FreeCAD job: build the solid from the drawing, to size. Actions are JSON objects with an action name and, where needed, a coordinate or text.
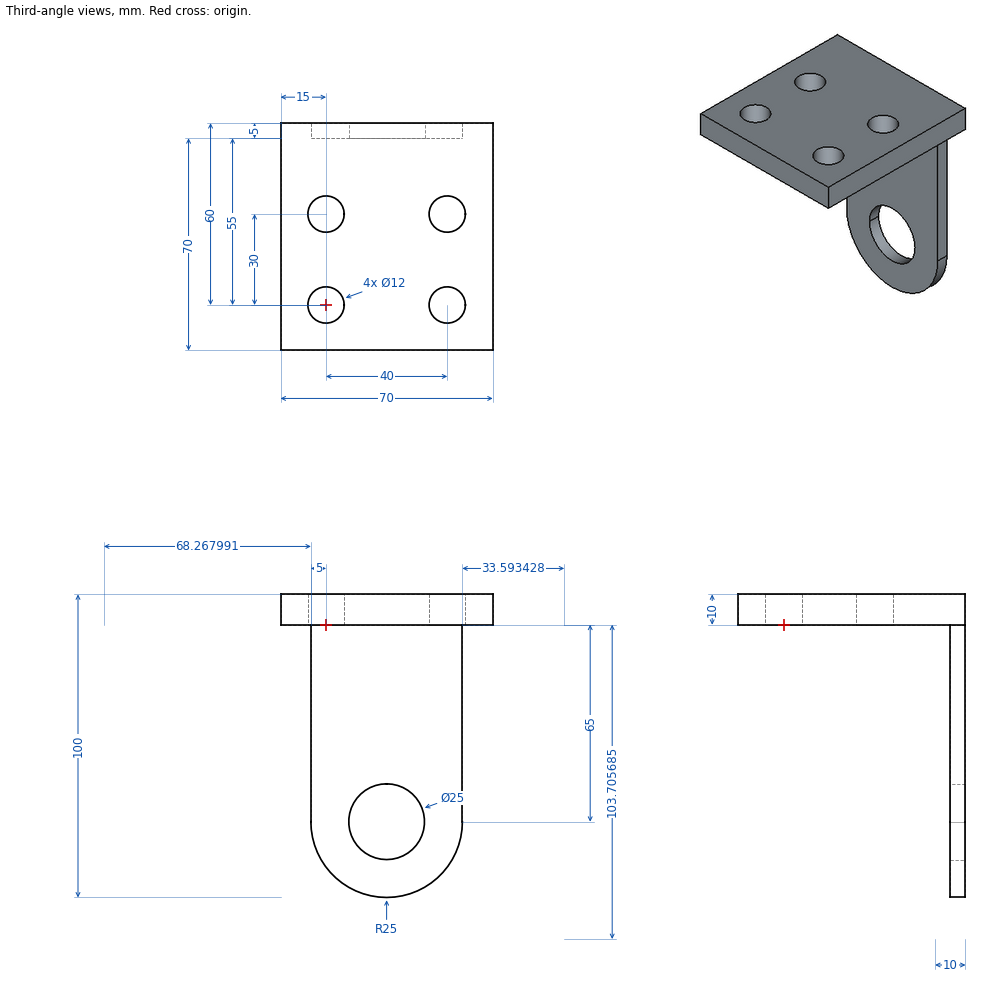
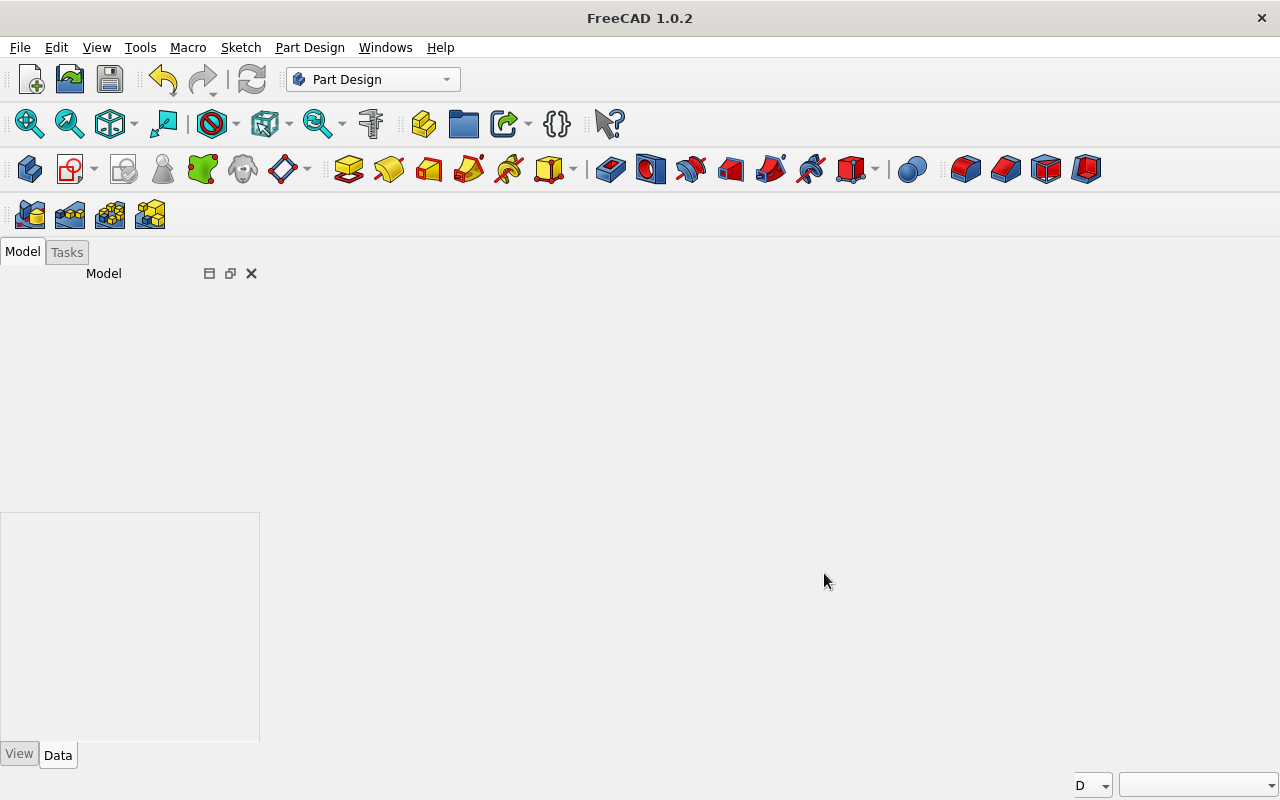
{"action": "left_click", "coordinate": [30, 80]}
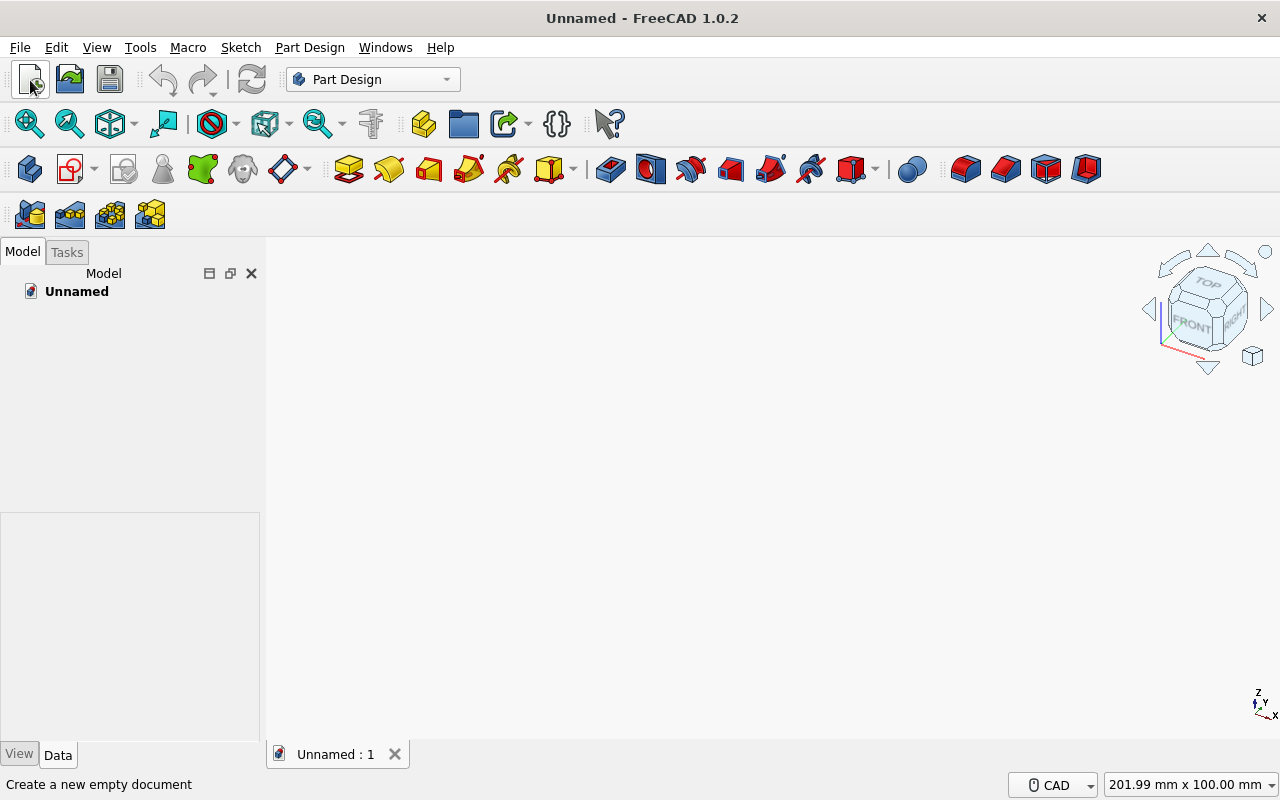
{"action": "left_click", "coordinate": [70, 170]}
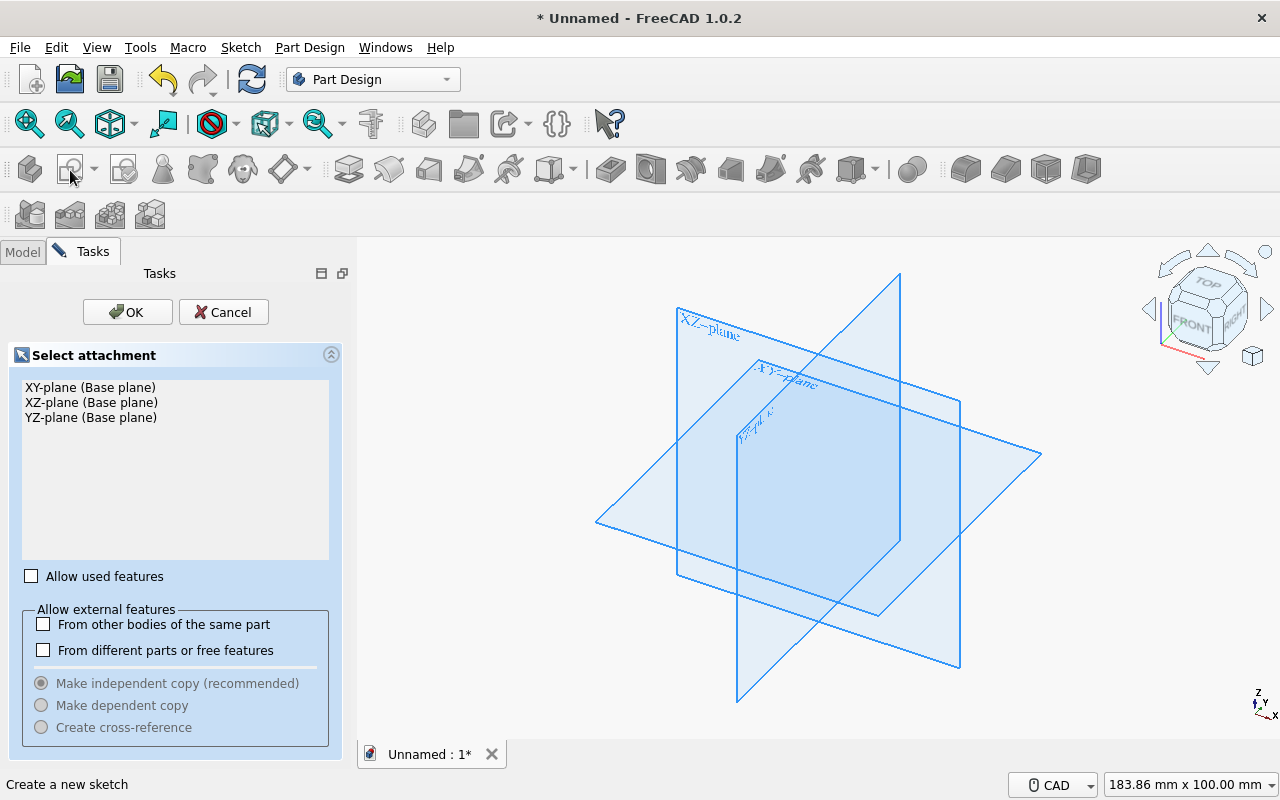
{"action": "left_click", "coordinate": [82, 388]}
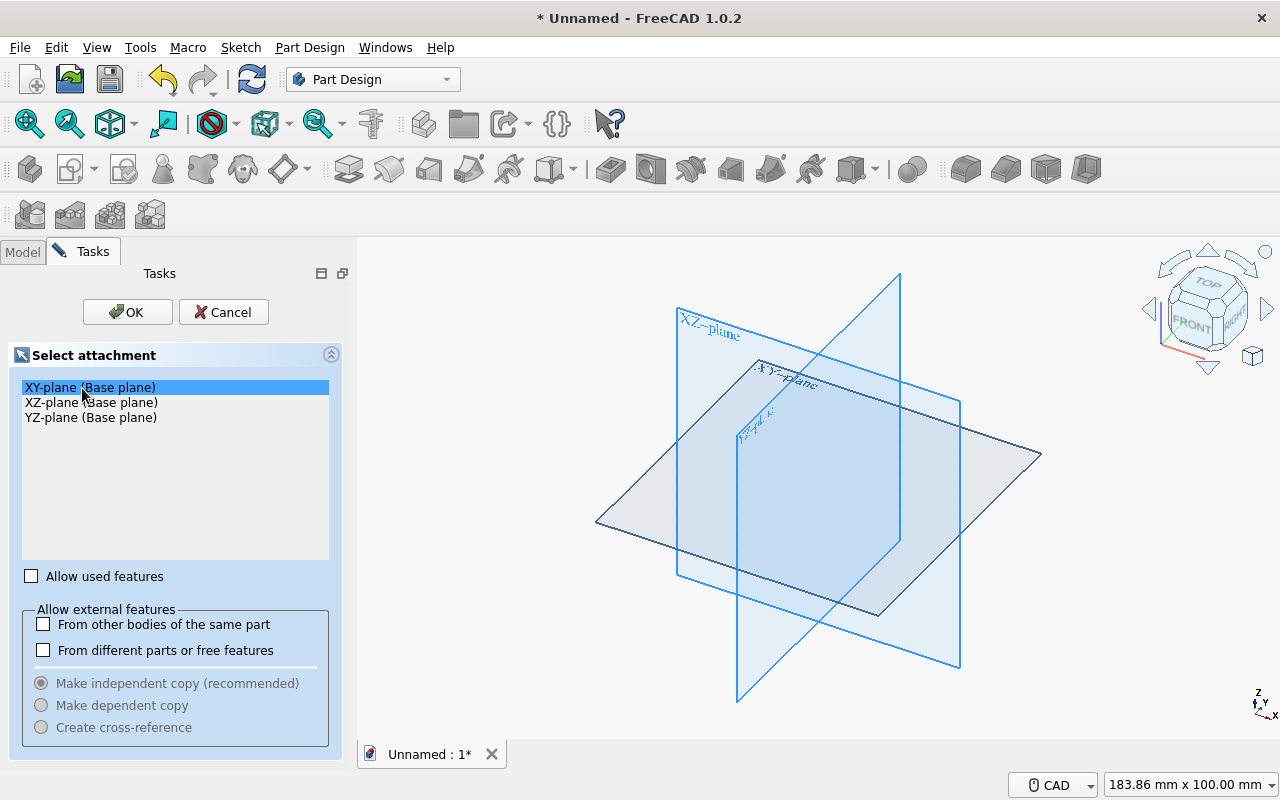
{"action": "left_click", "coordinate": [128, 312]}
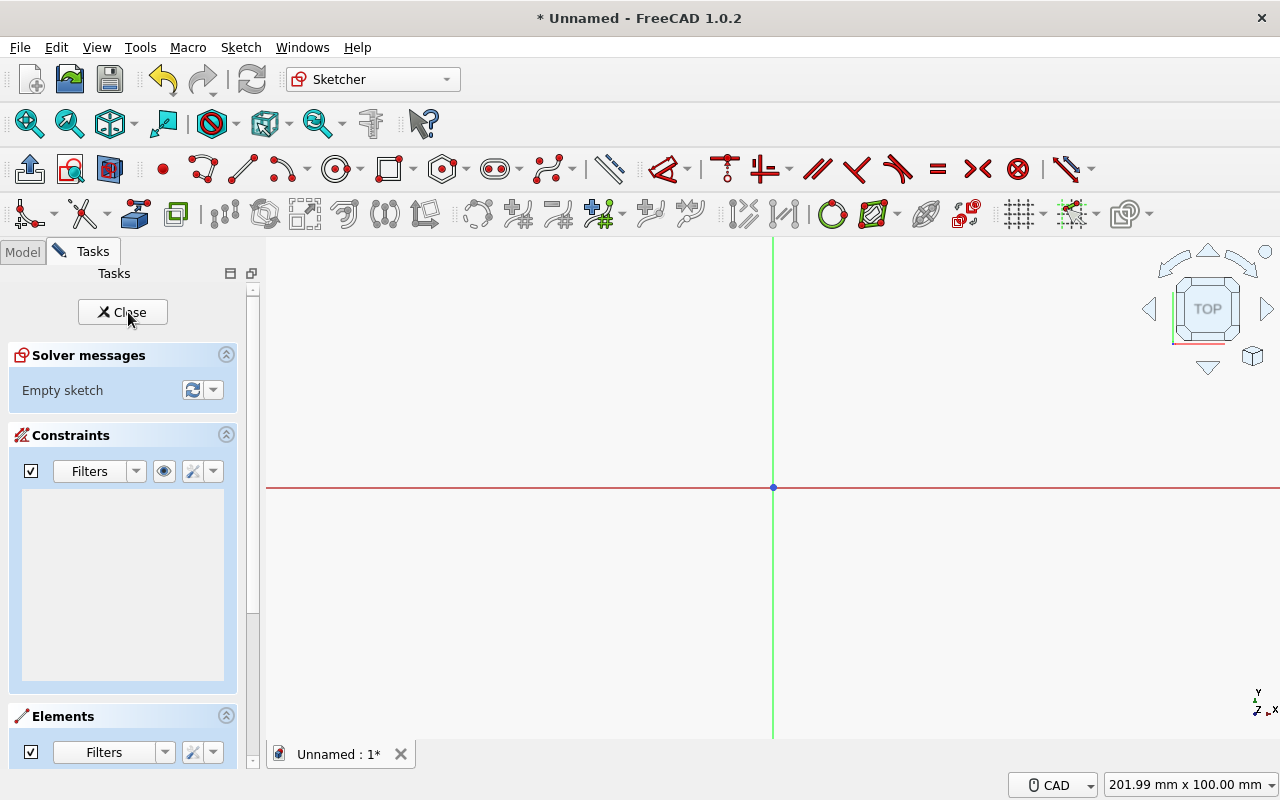
{"action": "scroll", "coordinate": [294, 711], "scroll_direction": "down", "scroll_amount": 1}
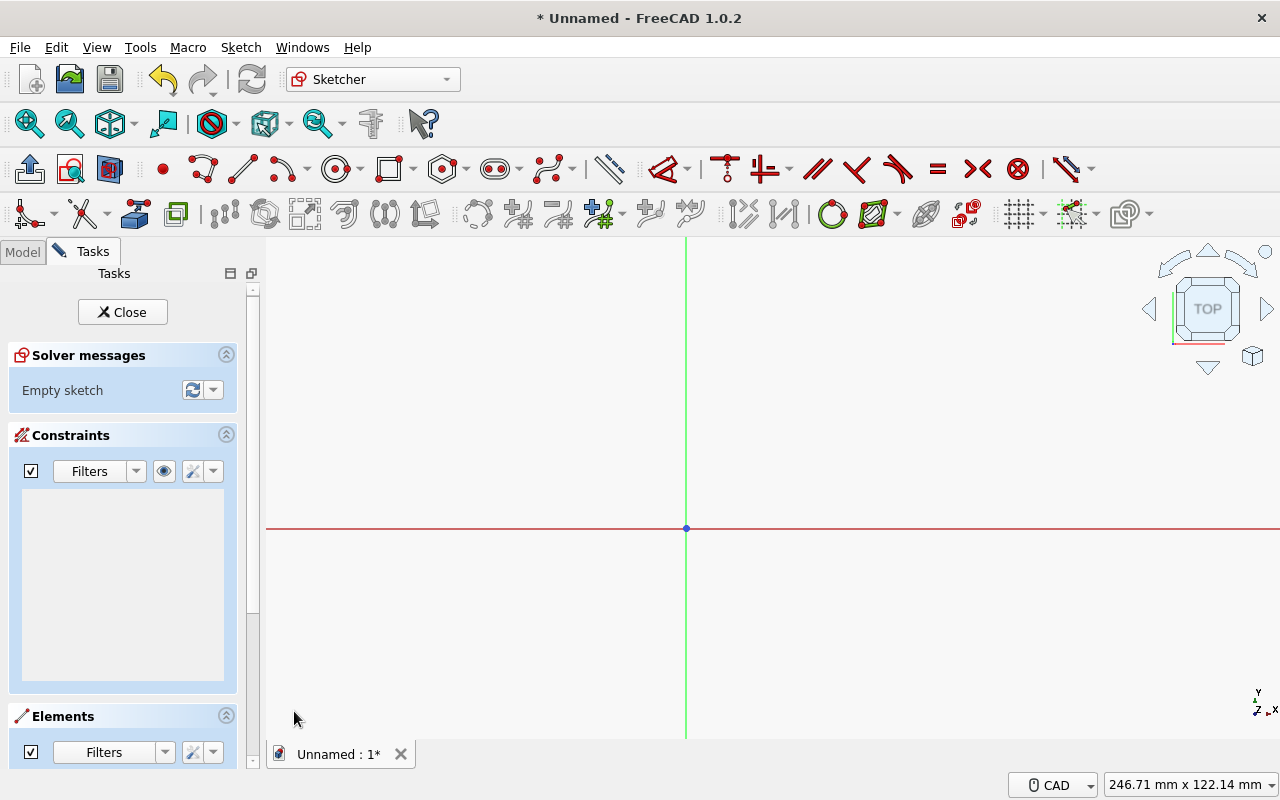
{"action": "left_click", "coordinate": [390, 170]}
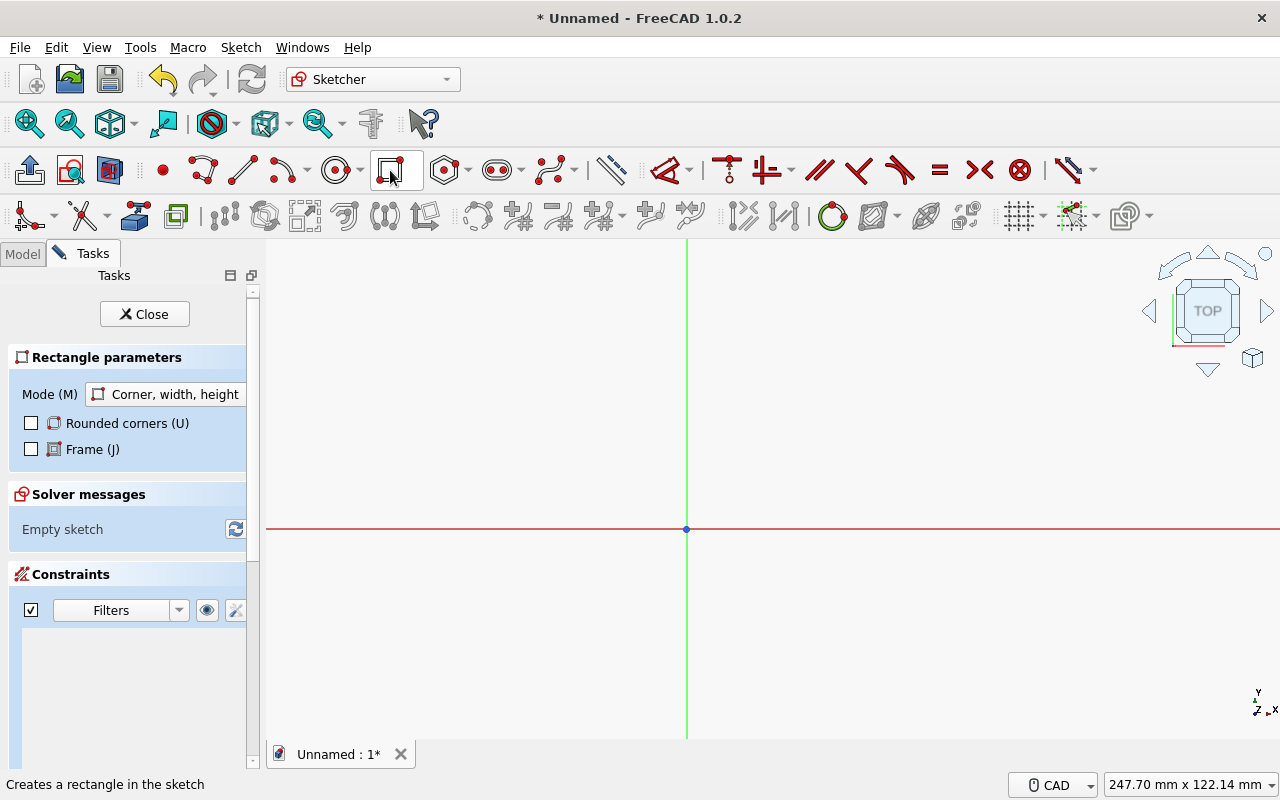
{"action": "left_click", "coordinate": [625, 304]}
{"action": "left_click", "coordinate": [912, 591]}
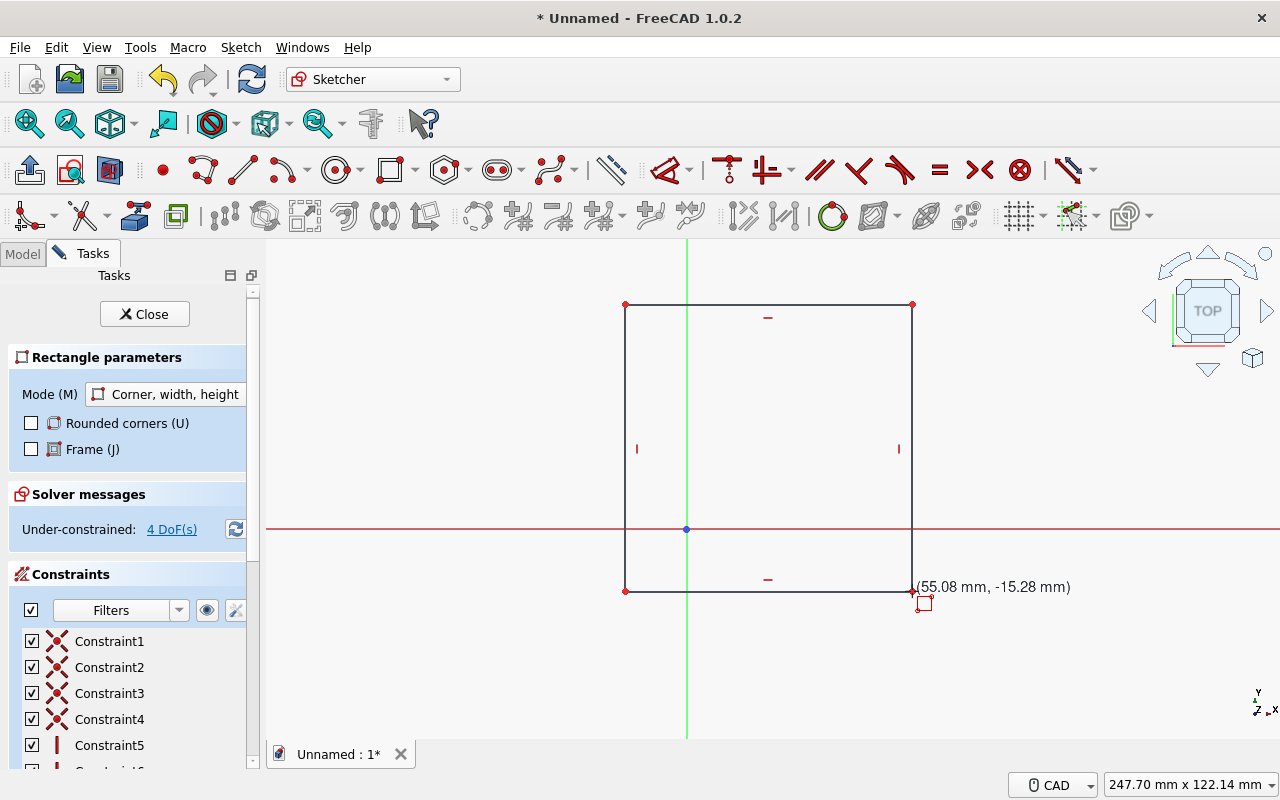
{"action": "left_click", "coordinate": [336, 170]}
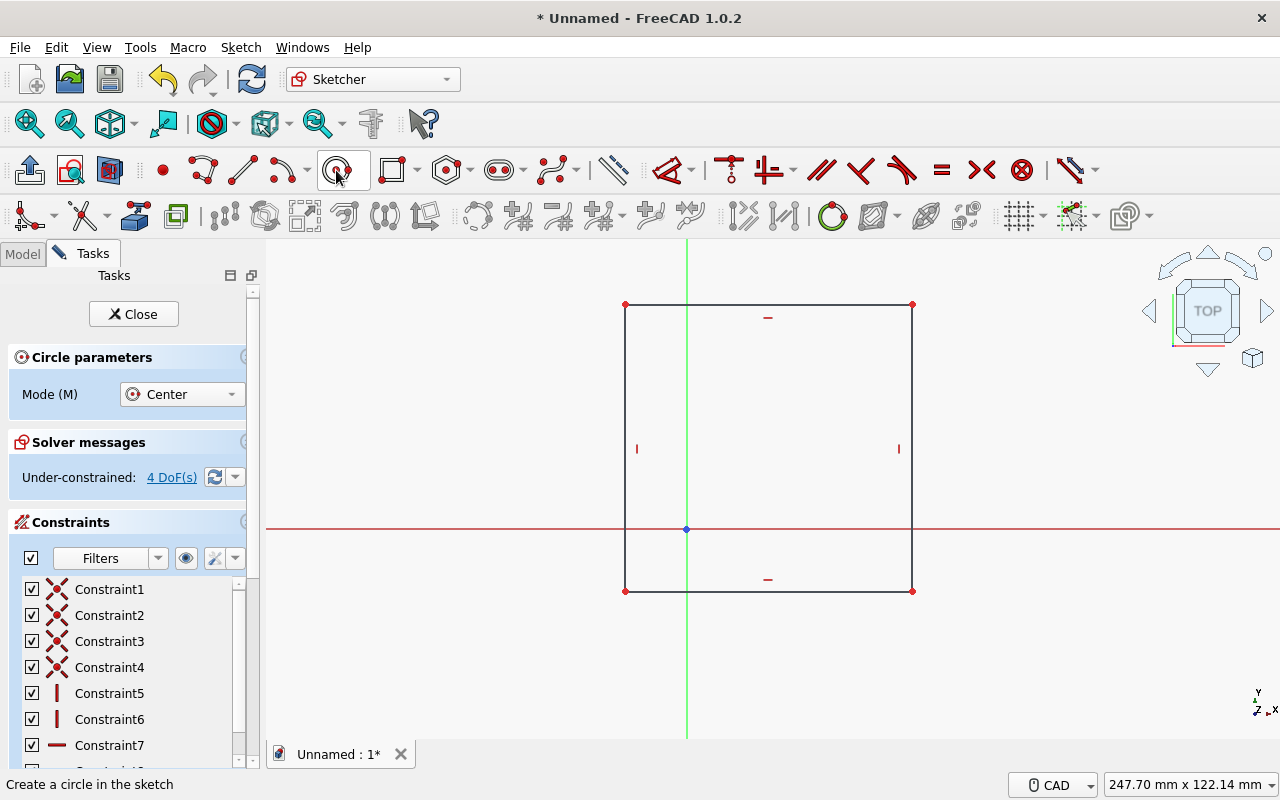
{"action": "left_click", "coordinate": [687, 529]}
{"action": "left_click", "coordinate": [704, 512]}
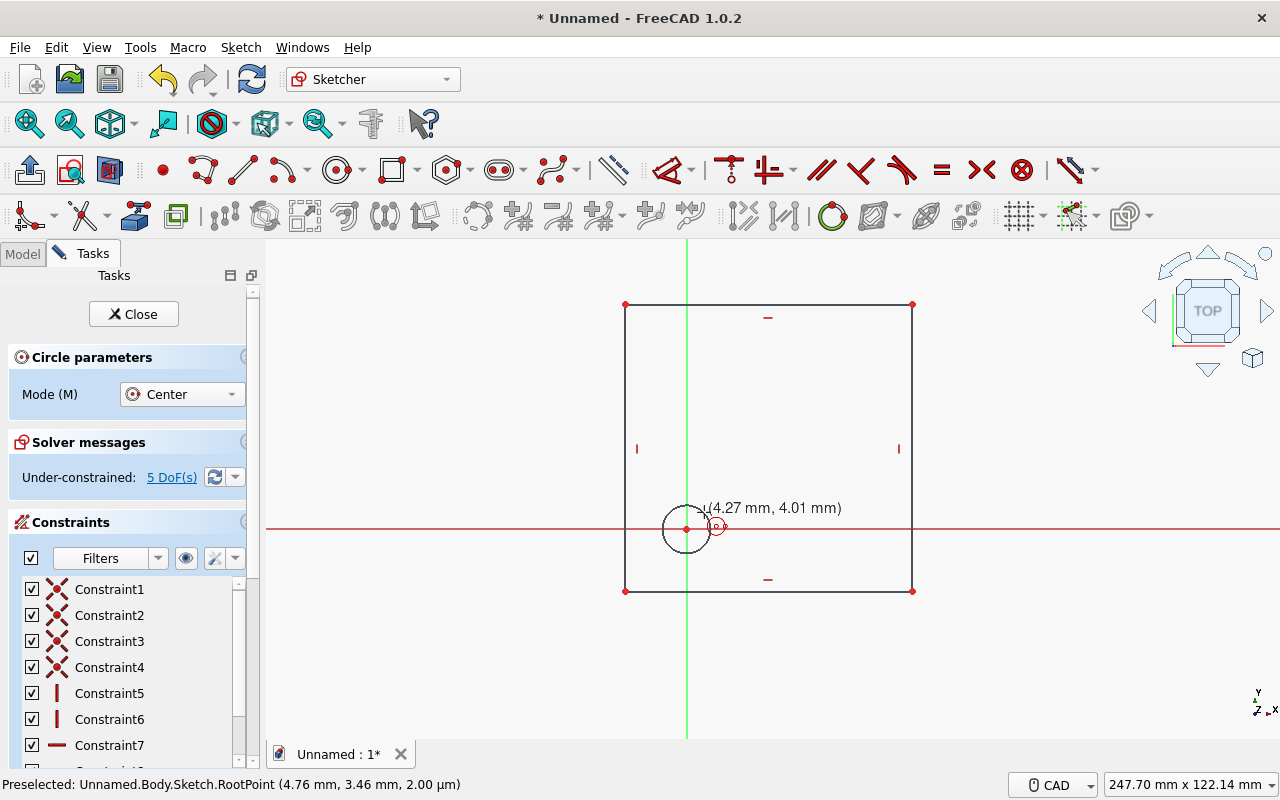
{"action": "left_click", "coordinate": [850, 529]}
{"action": "left_click", "coordinate": [868, 512]}